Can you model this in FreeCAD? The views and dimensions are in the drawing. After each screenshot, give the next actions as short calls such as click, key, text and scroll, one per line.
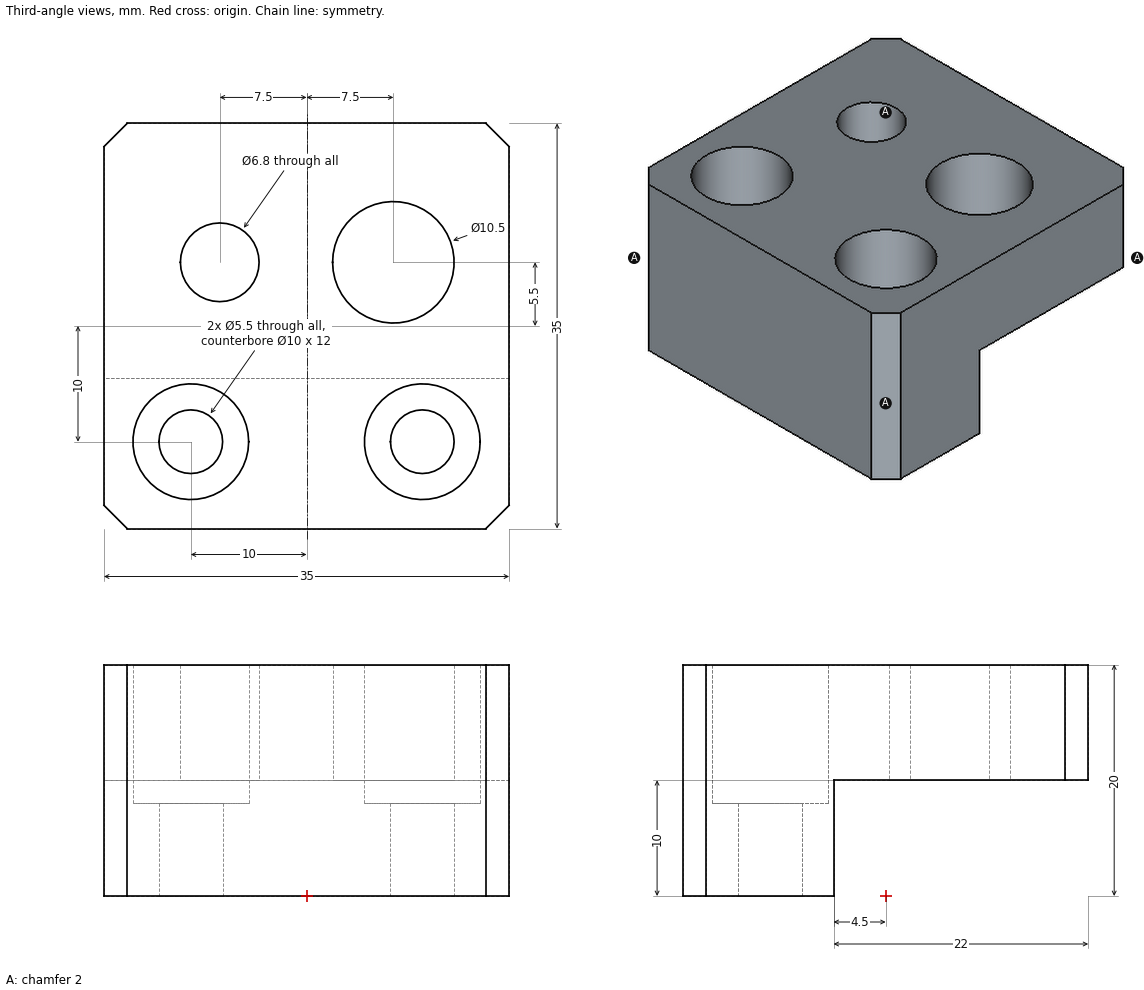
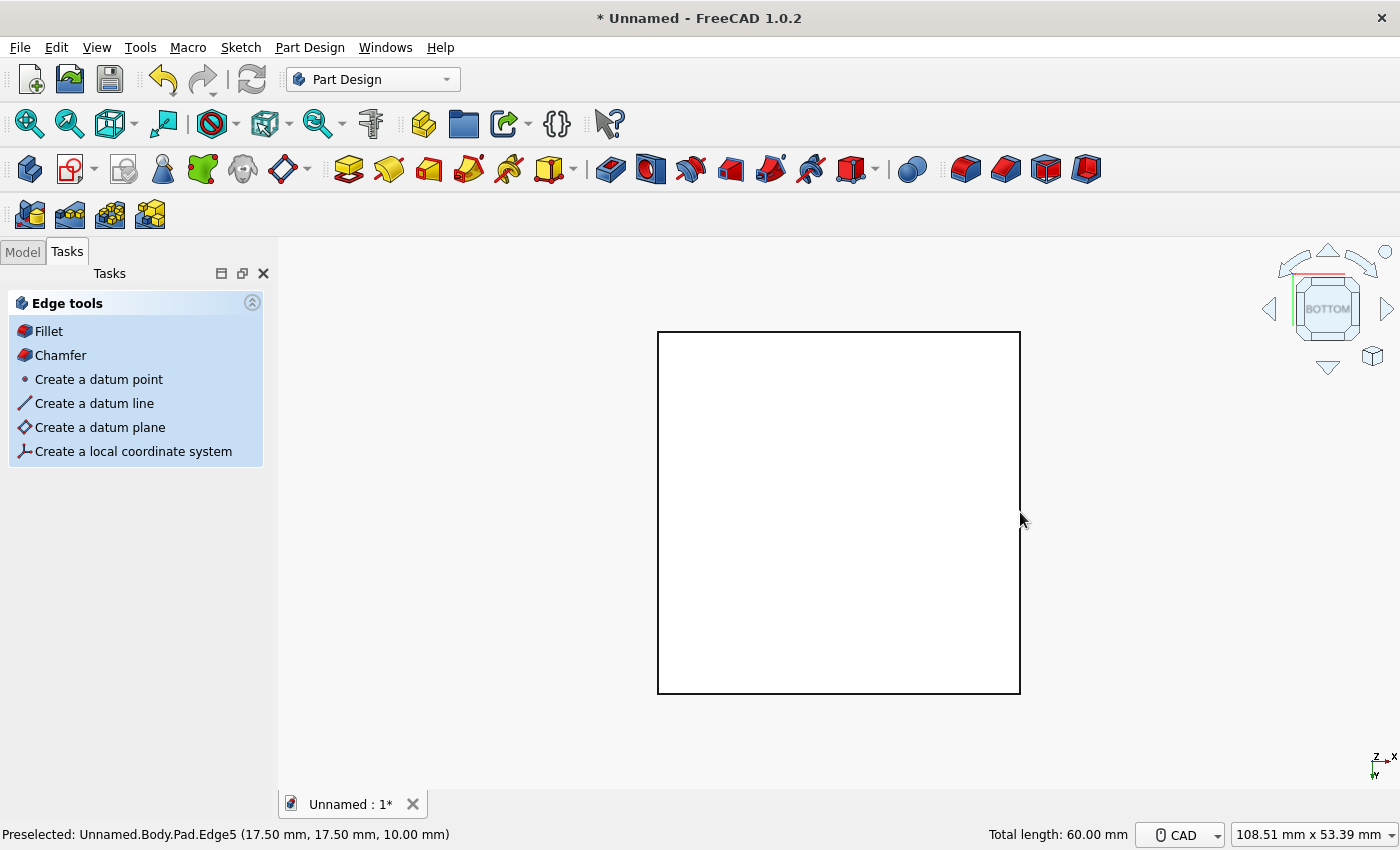
key(4)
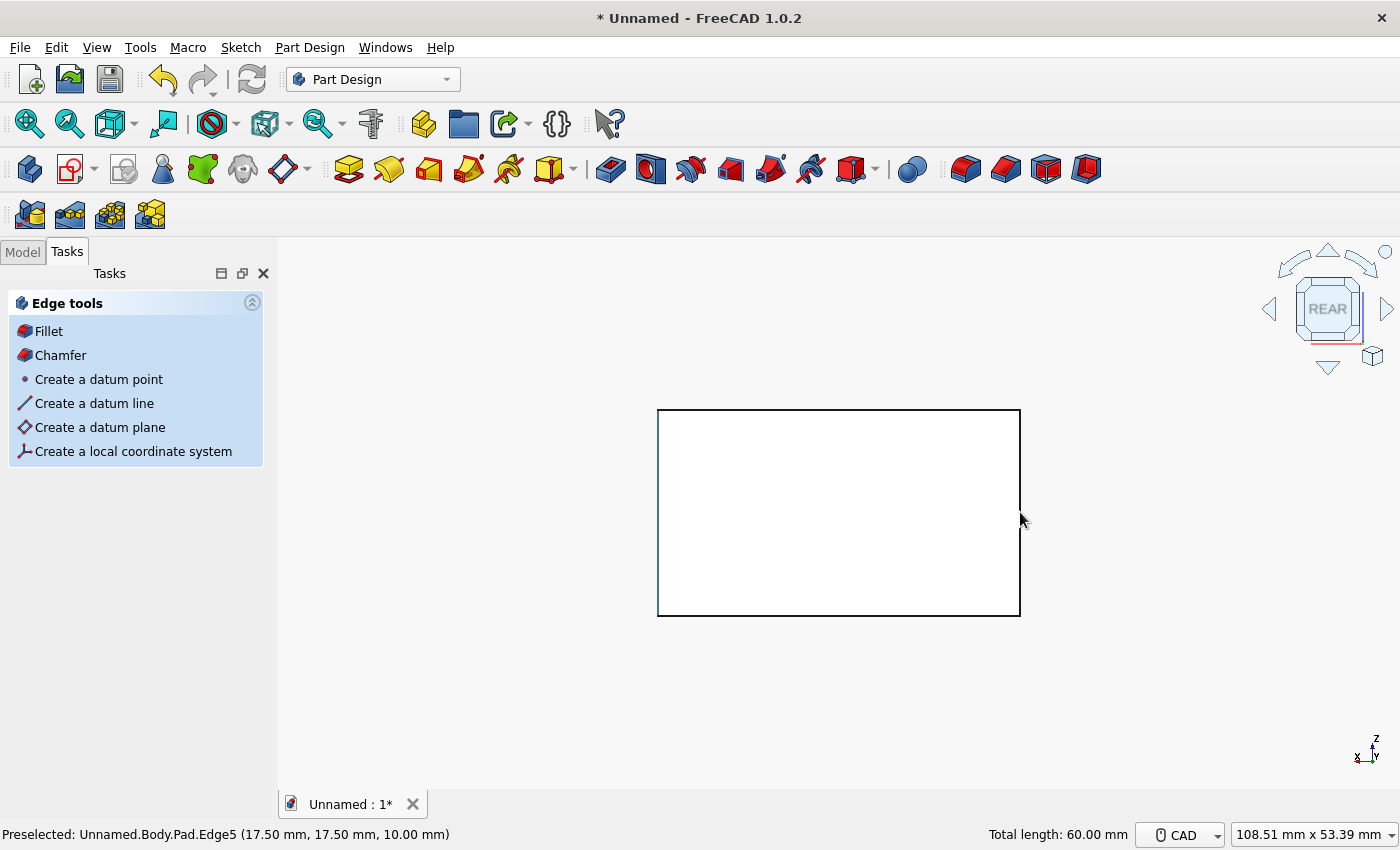
key(v)
key(f)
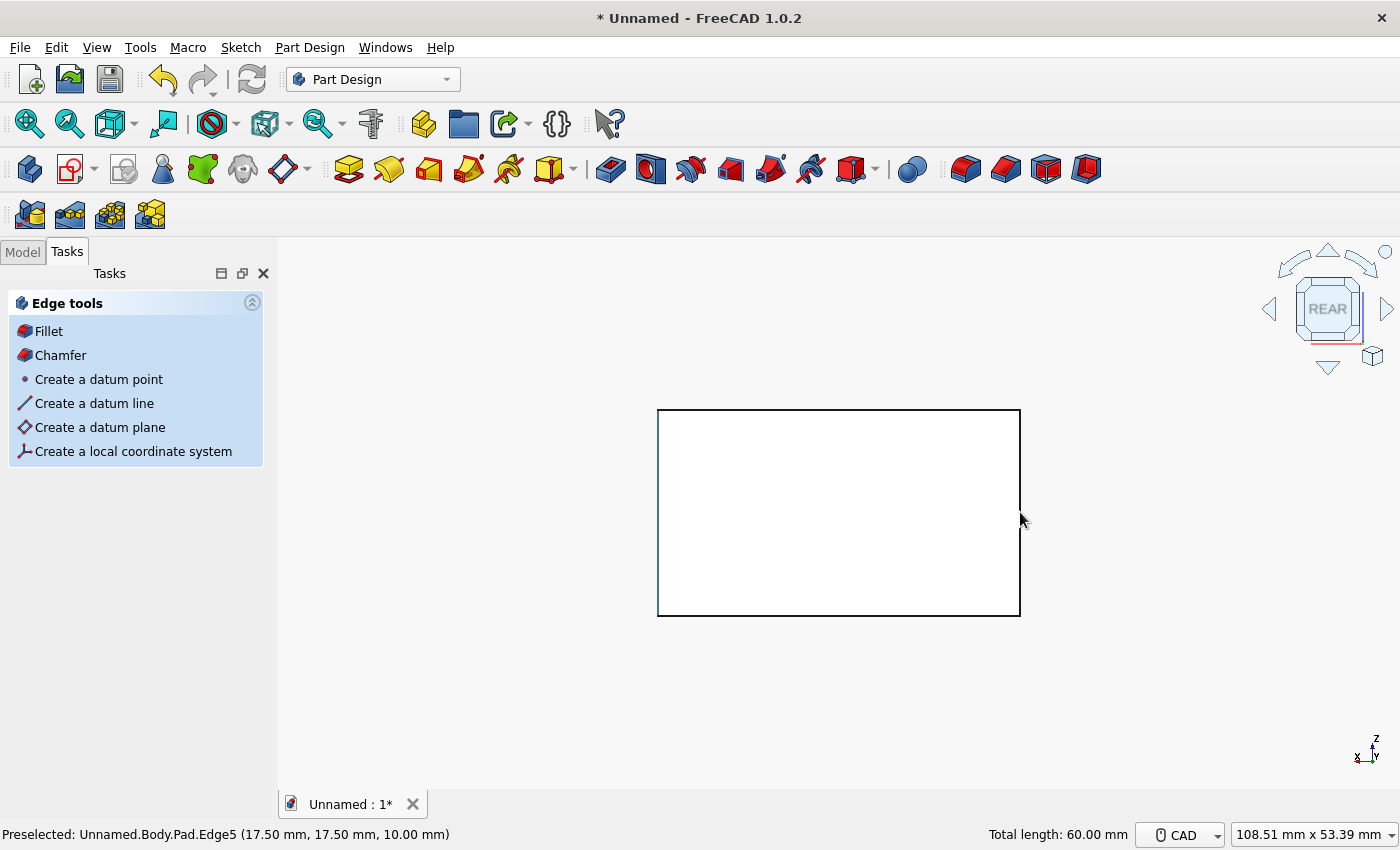
click(1020, 512, ctrl)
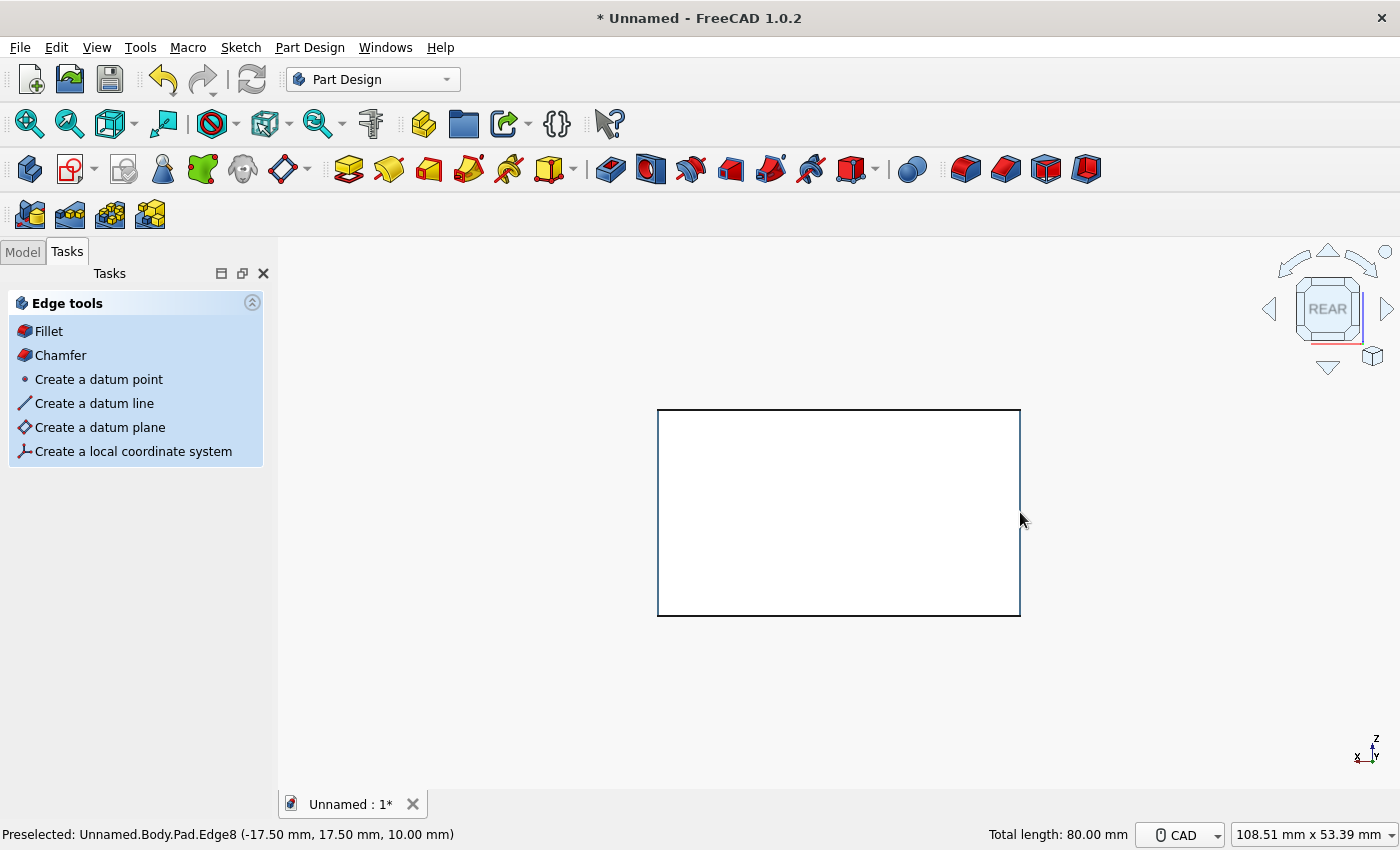
click(1006, 170)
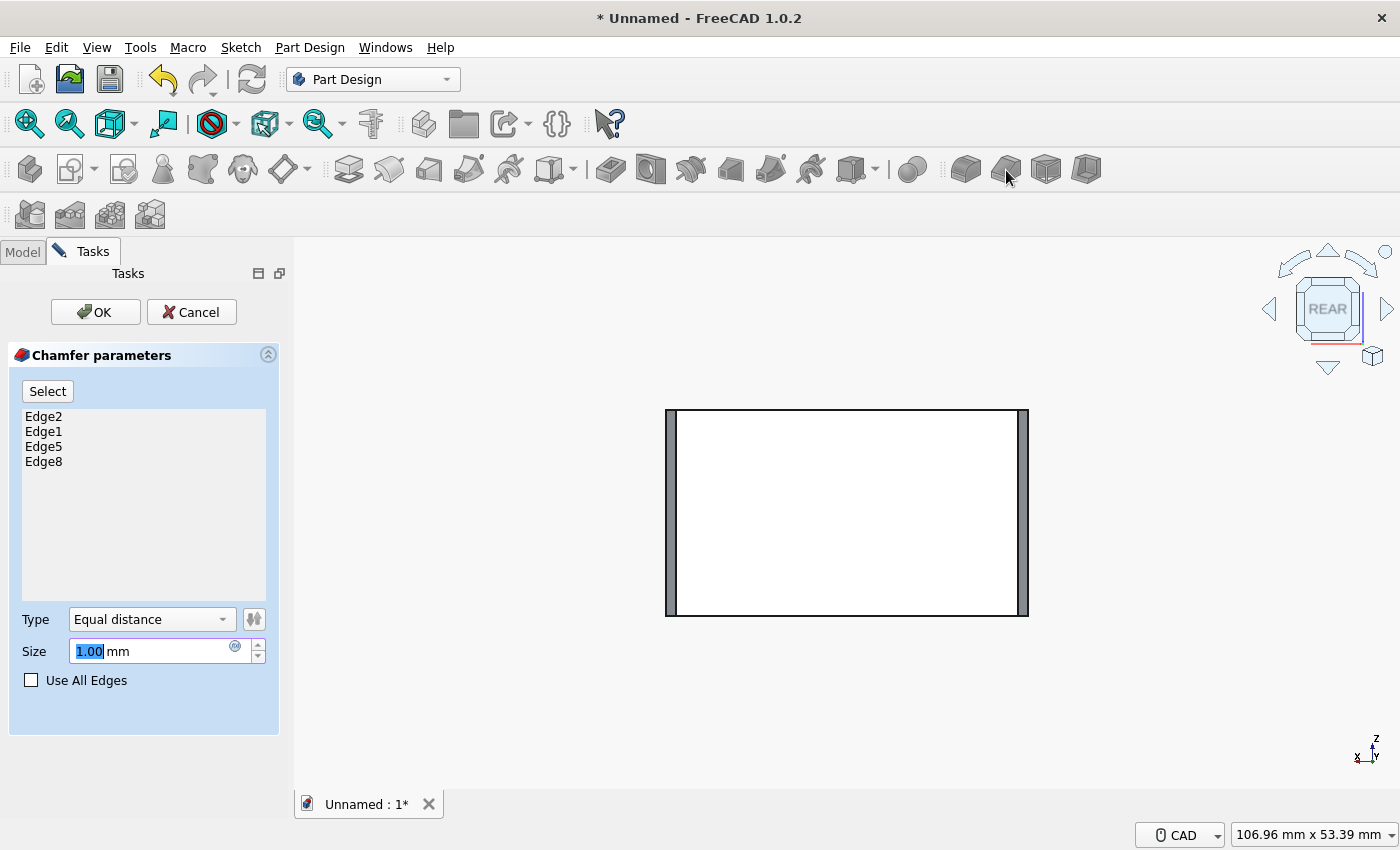
text(2)
key(Tab)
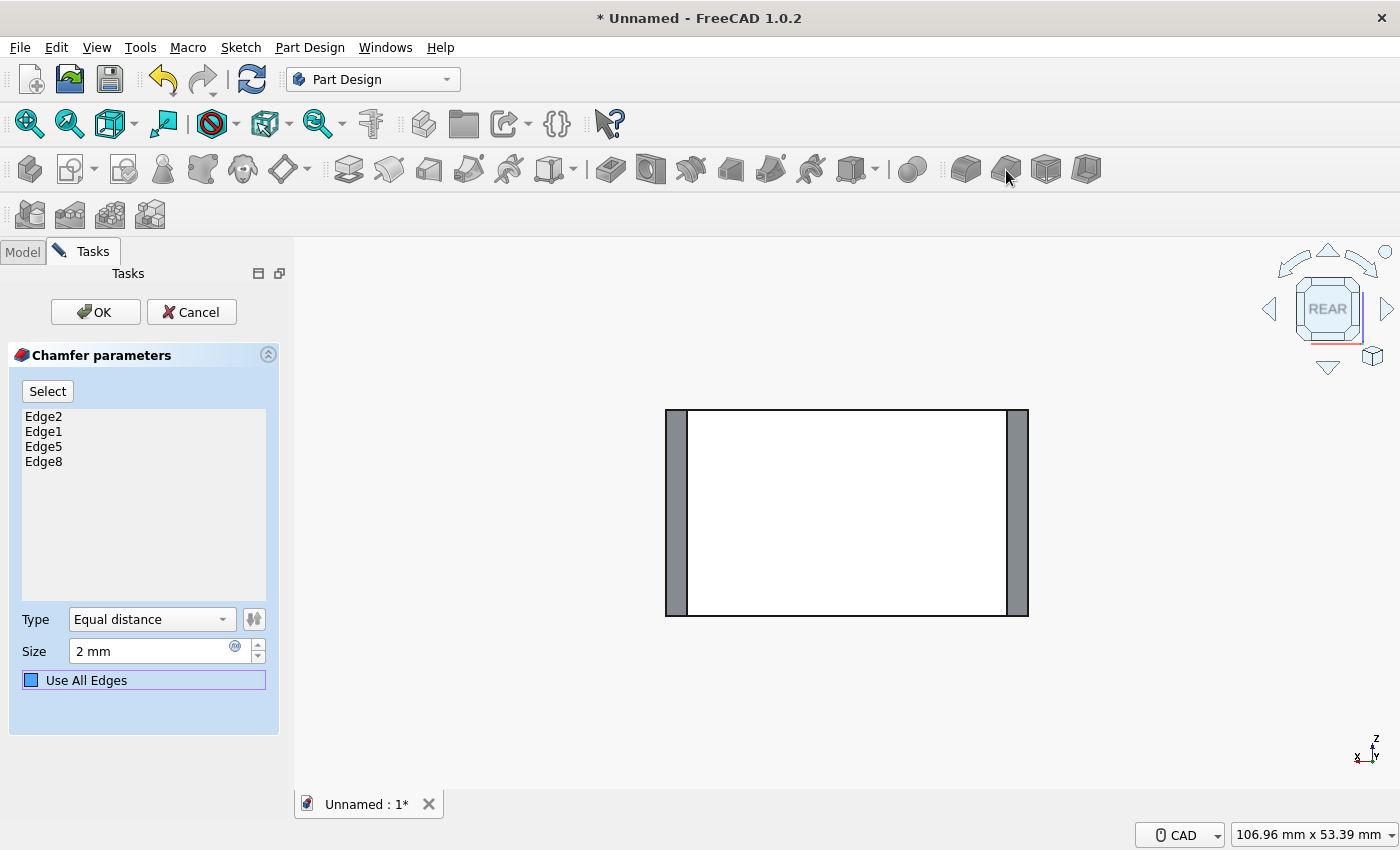
click(96, 312)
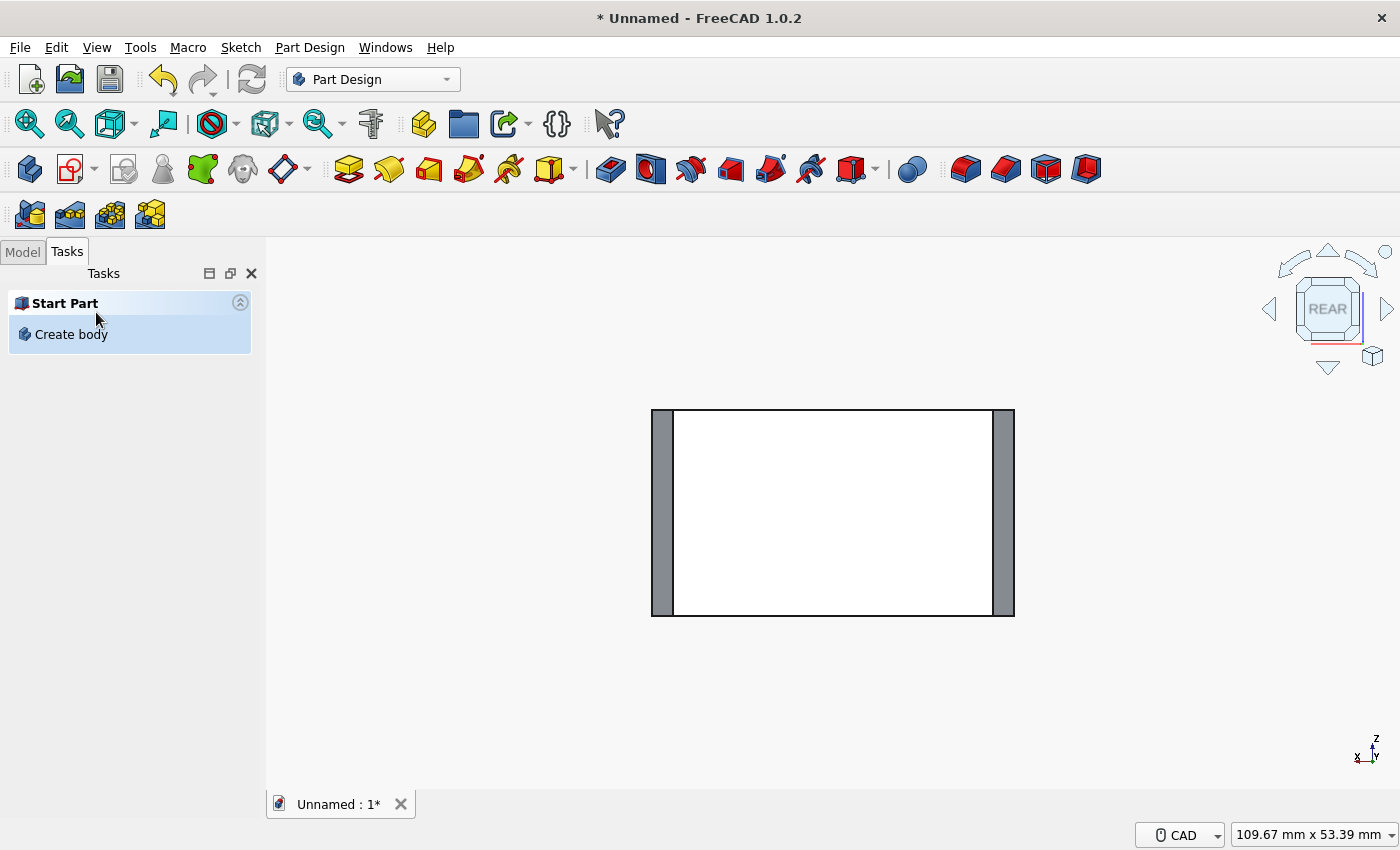
click(30, 124)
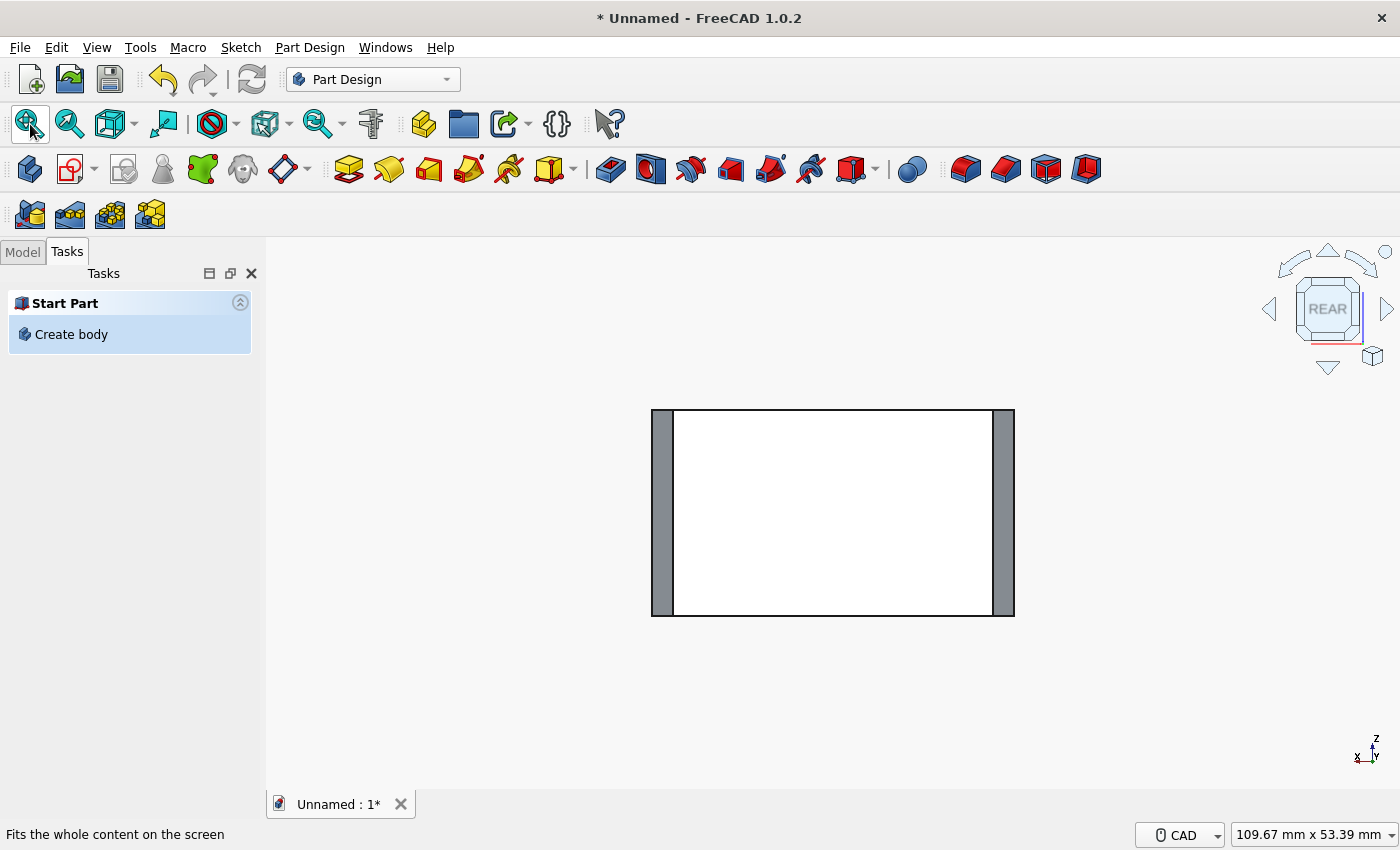
key(0)